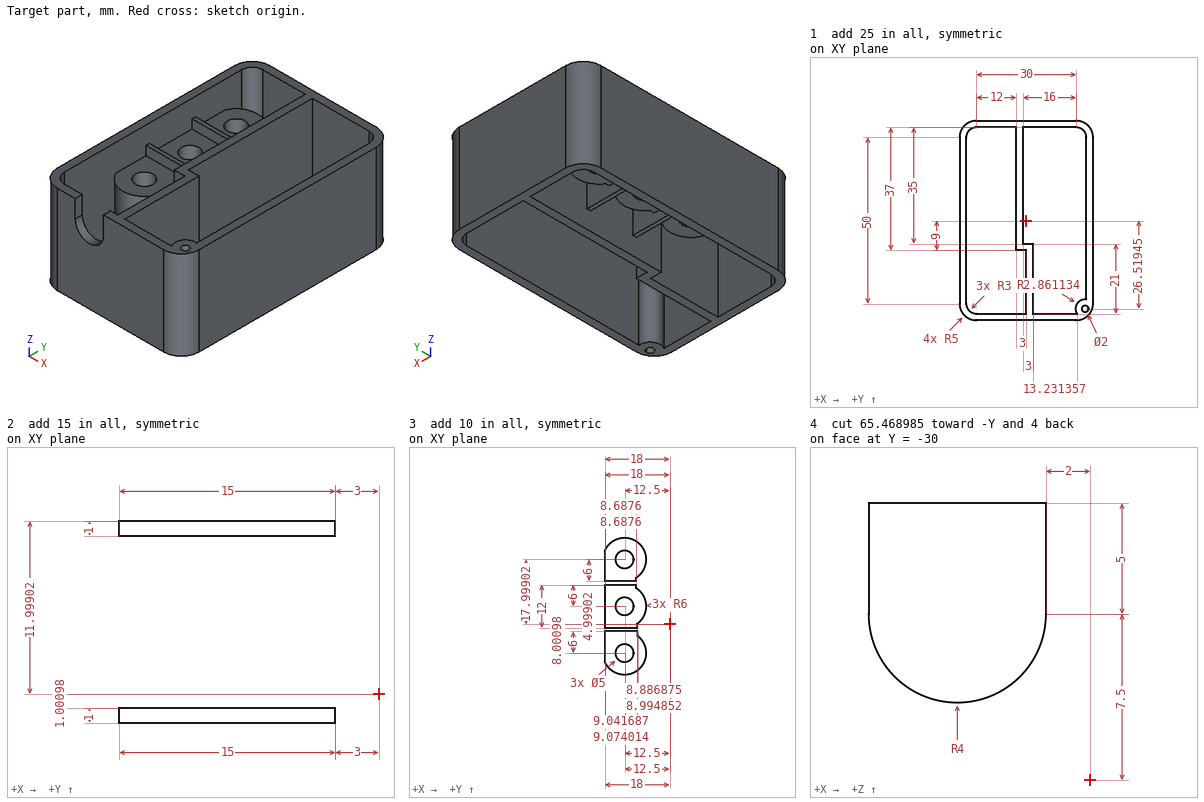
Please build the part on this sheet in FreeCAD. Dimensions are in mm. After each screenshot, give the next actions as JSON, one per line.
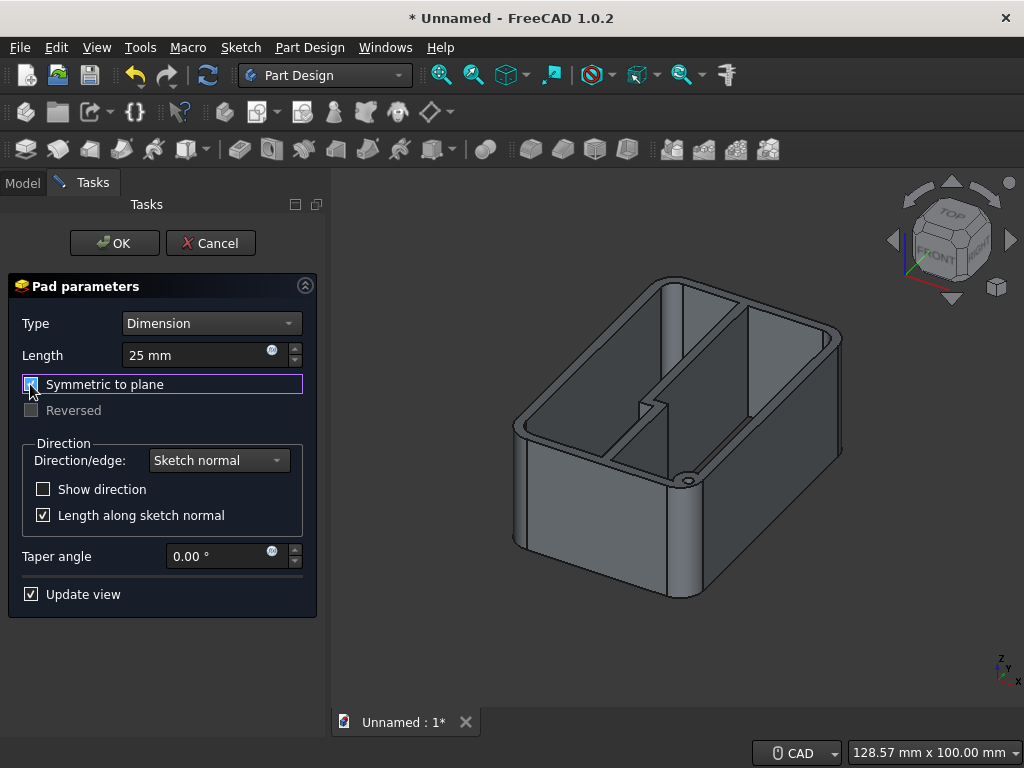
{"action": "left_click", "coordinate": [115, 243]}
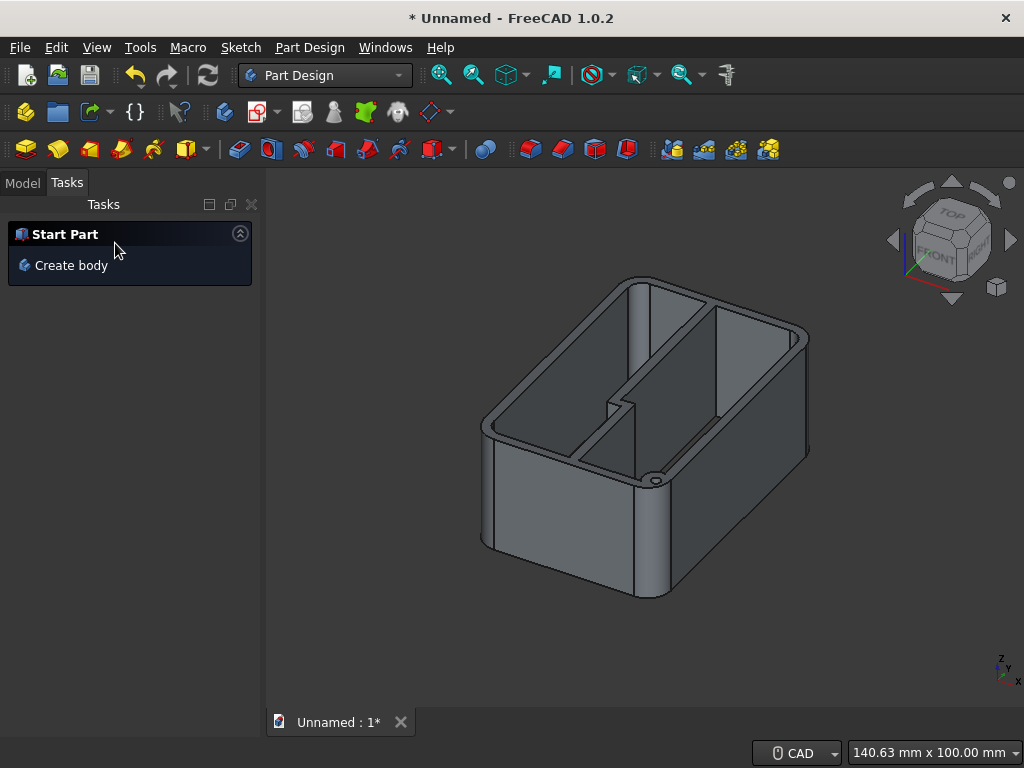
{"action": "left_click", "coordinate": [258, 112]}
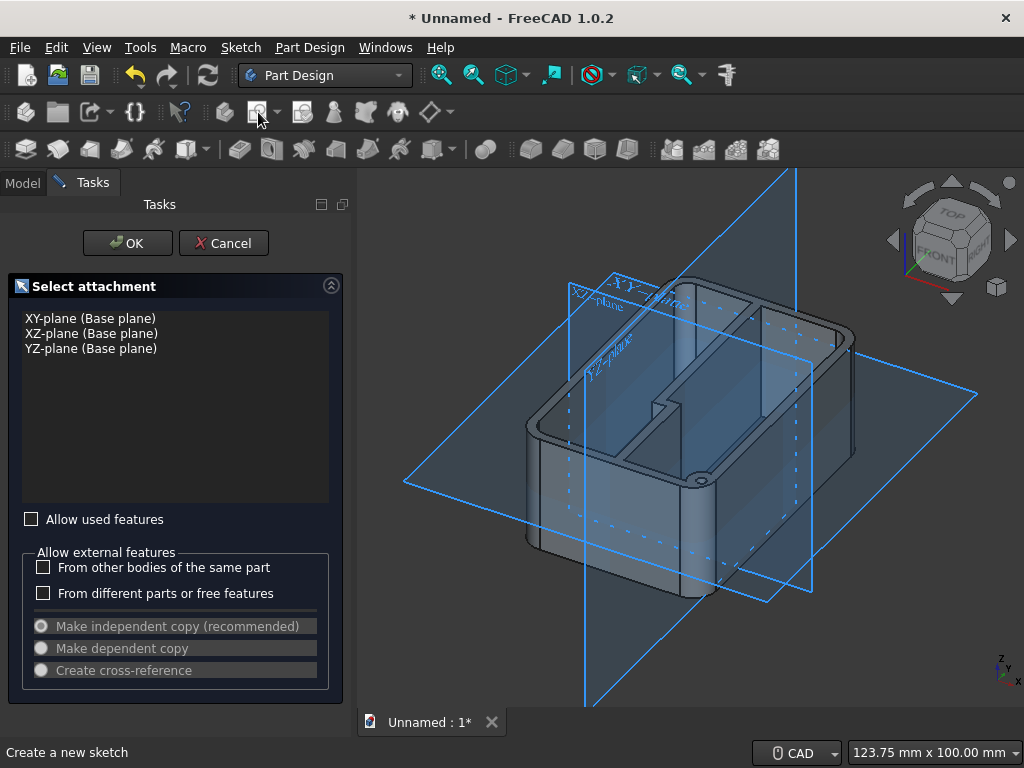
{"action": "left_click", "coordinate": [82, 318]}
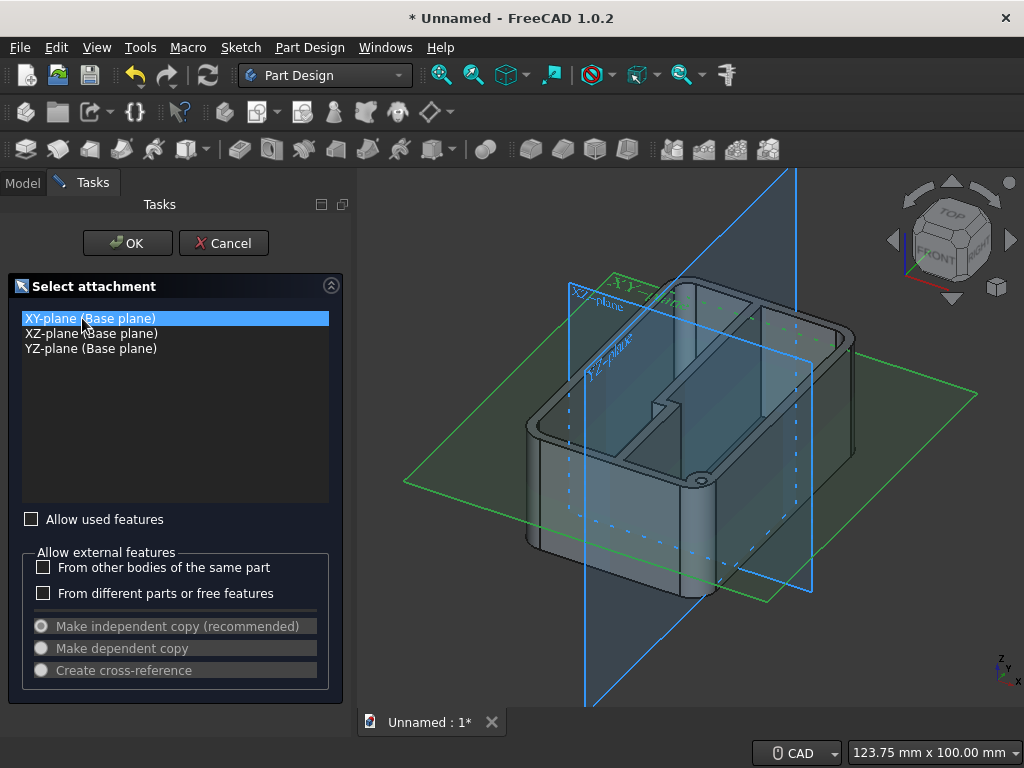
{"action": "left_click", "coordinate": [128, 243]}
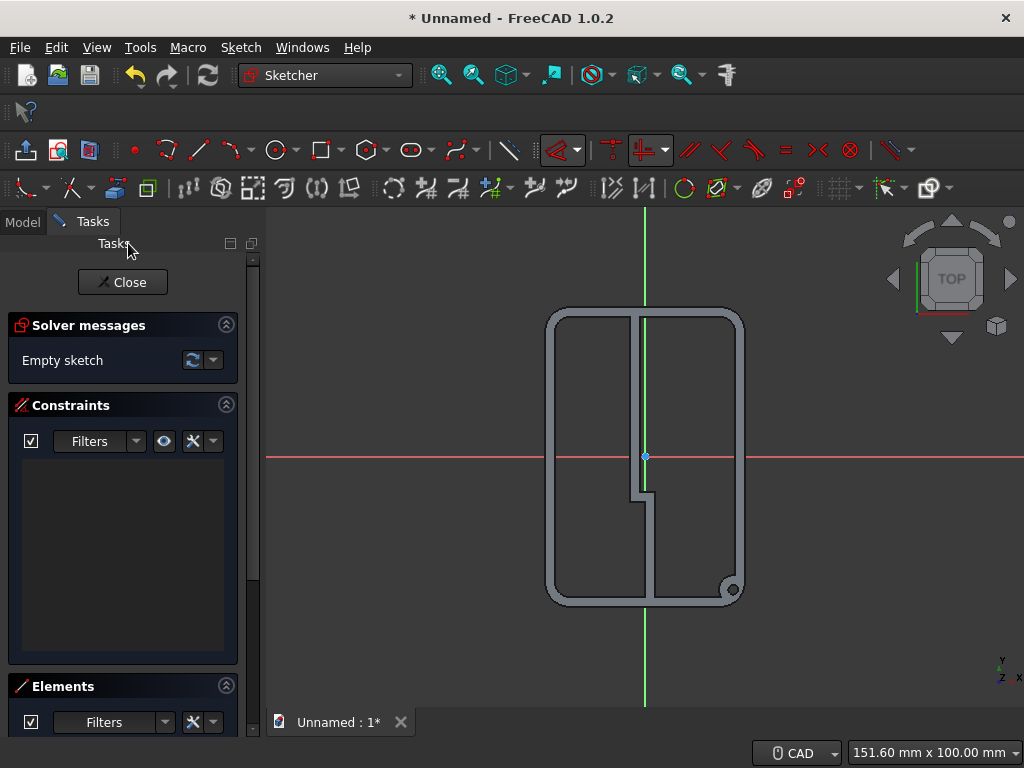
{"action": "left_click", "coordinate": [90, 150]}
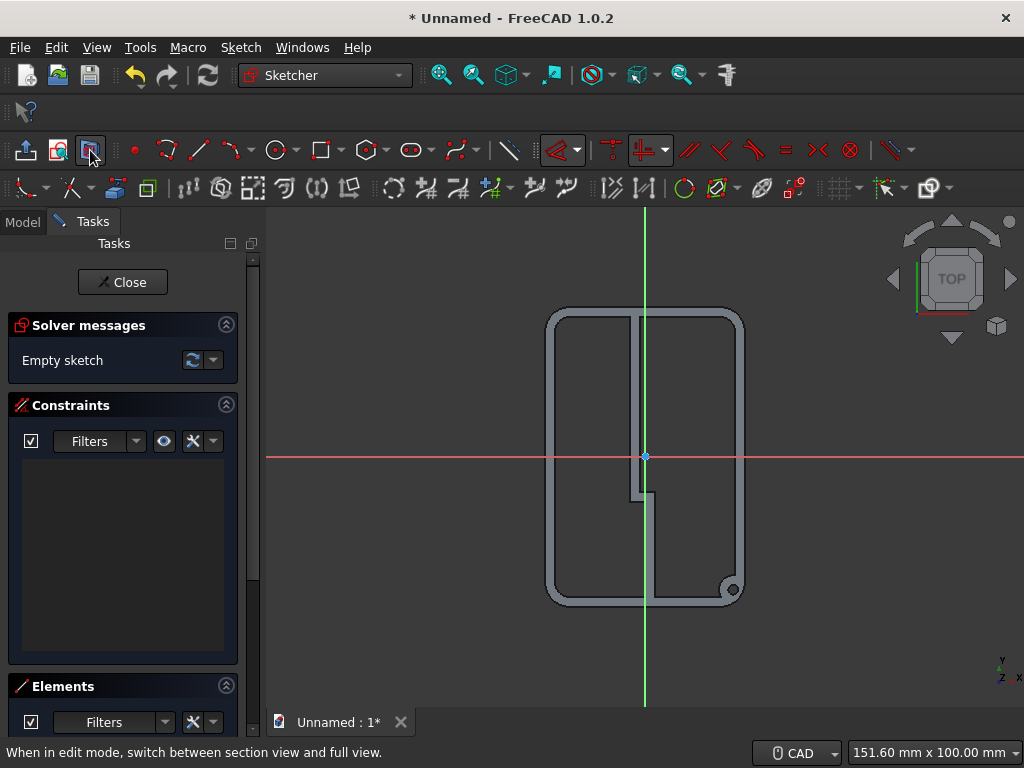
{"action": "scroll", "coordinate": [608, 424], "scroll_direction": "up", "scroll_amount": 7}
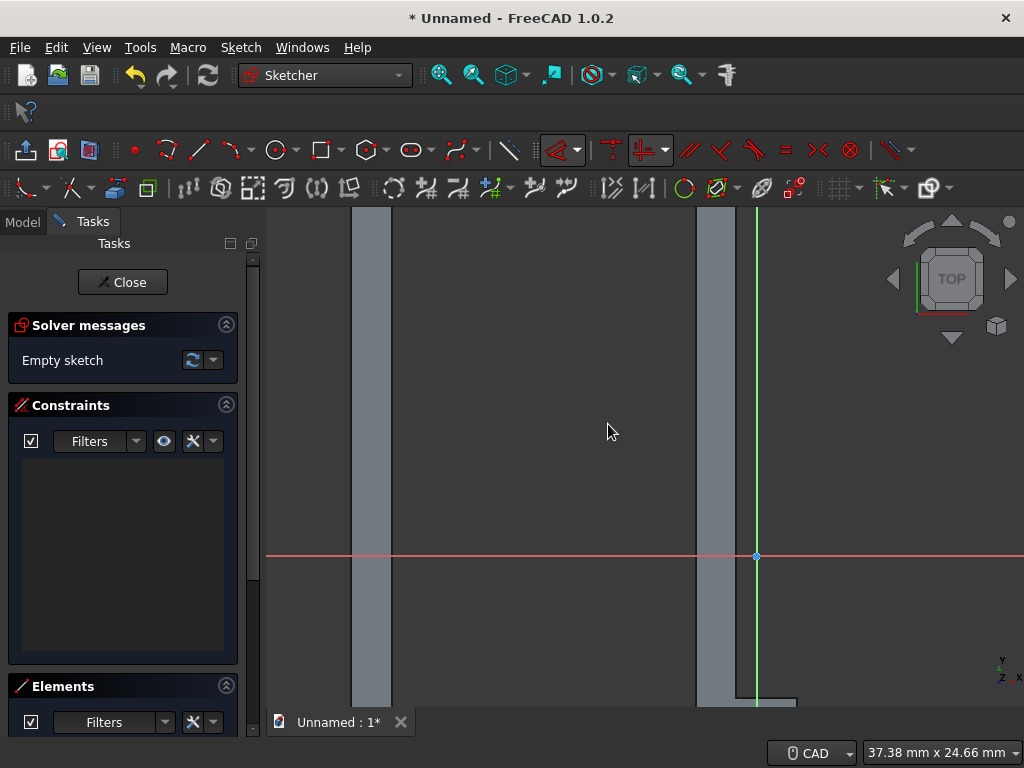
{"action": "left_click", "coordinate": [322, 150]}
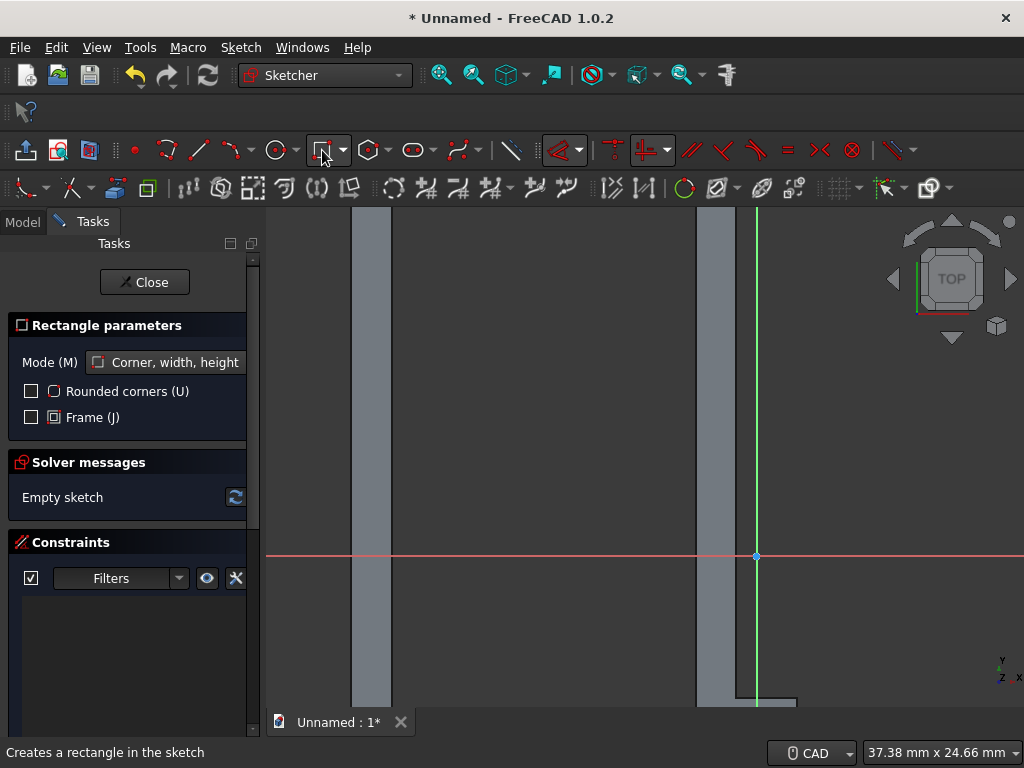
{"action": "left_click", "coordinate": [392, 577]}
{"action": "left_click", "coordinate": [696, 597]}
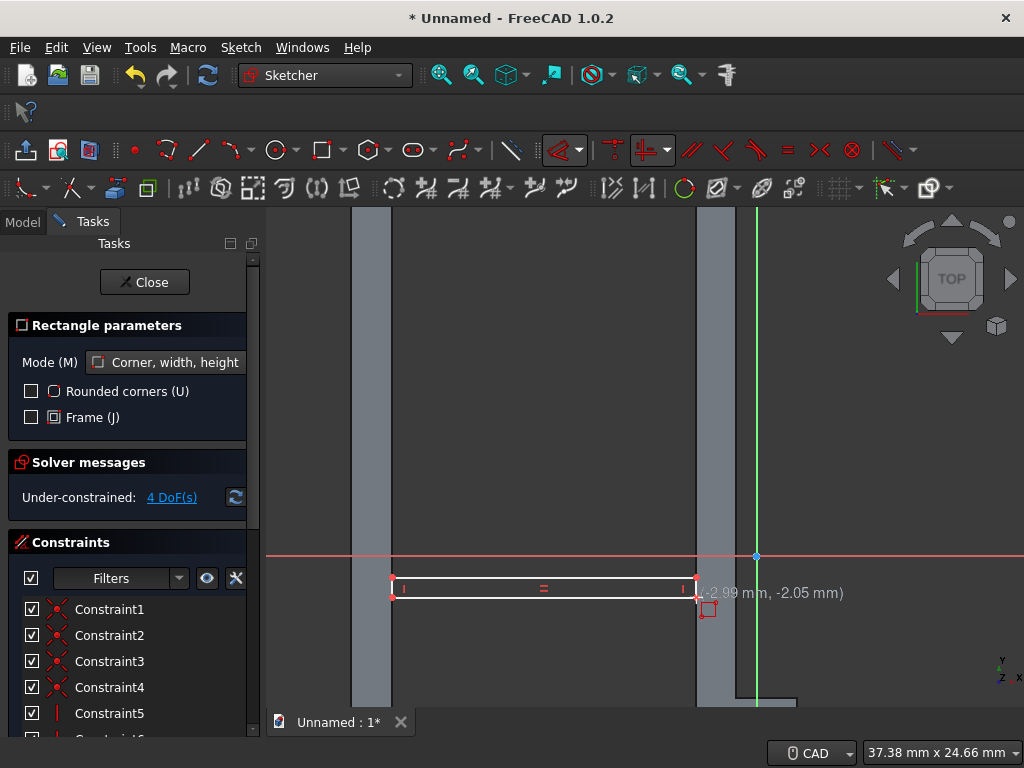
{"action": "left_click", "coordinate": [392, 313]}
{"action": "left_click", "coordinate": [696, 333]}
{"action": "key", "text": "Escape"}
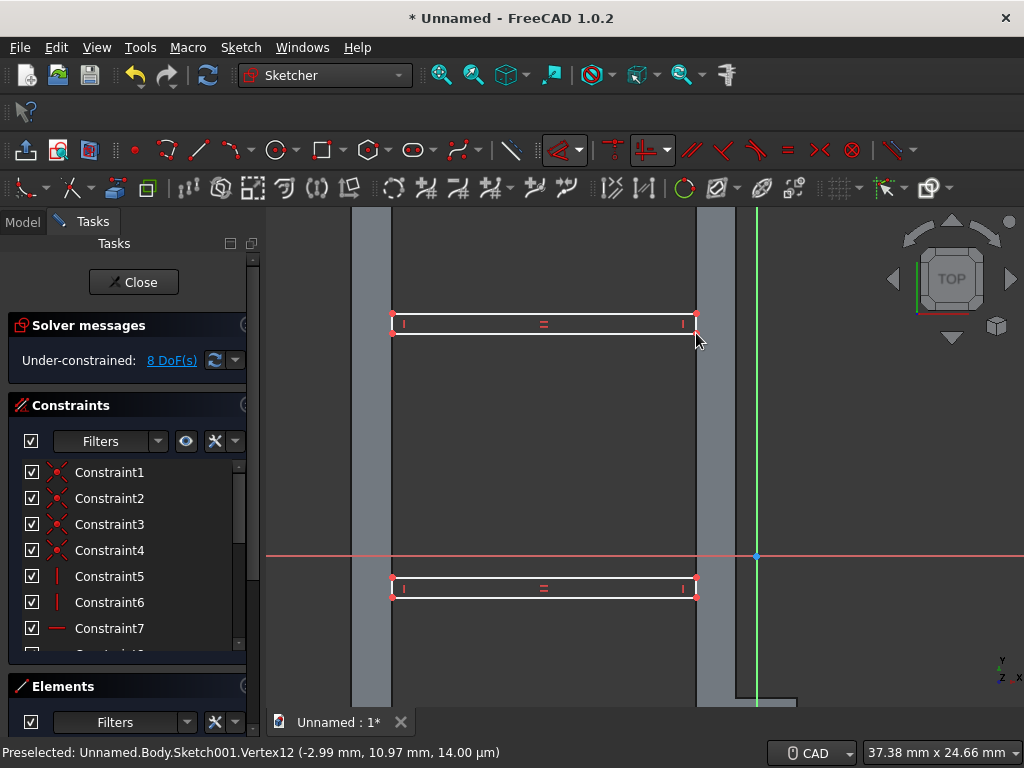
{"action": "scroll", "coordinate": [392, 588], "scroll_direction": "up", "scroll_amount": 4}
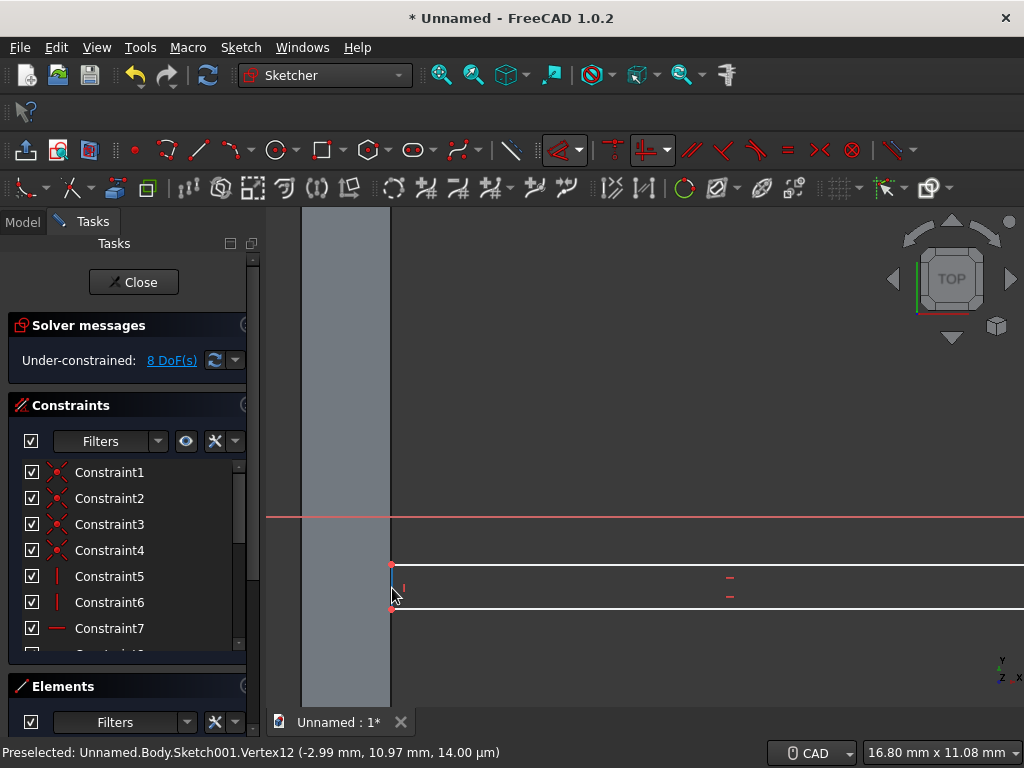
{"action": "left_click", "coordinate": [392, 587]}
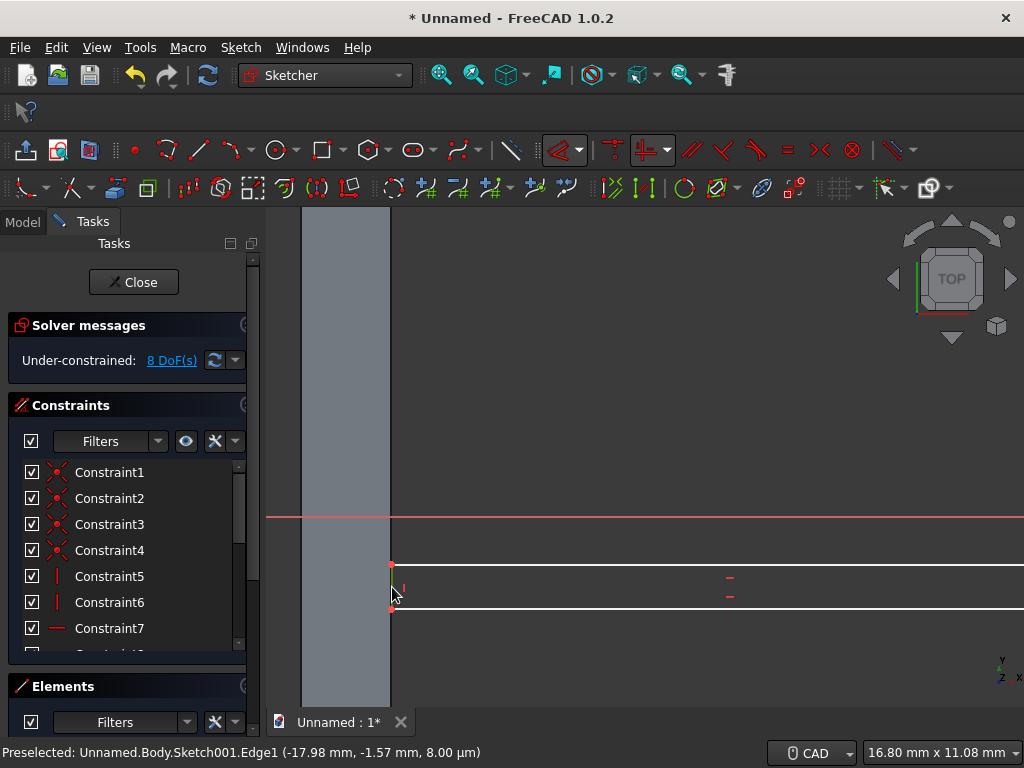
{"action": "left_click", "coordinate": [582, 150]}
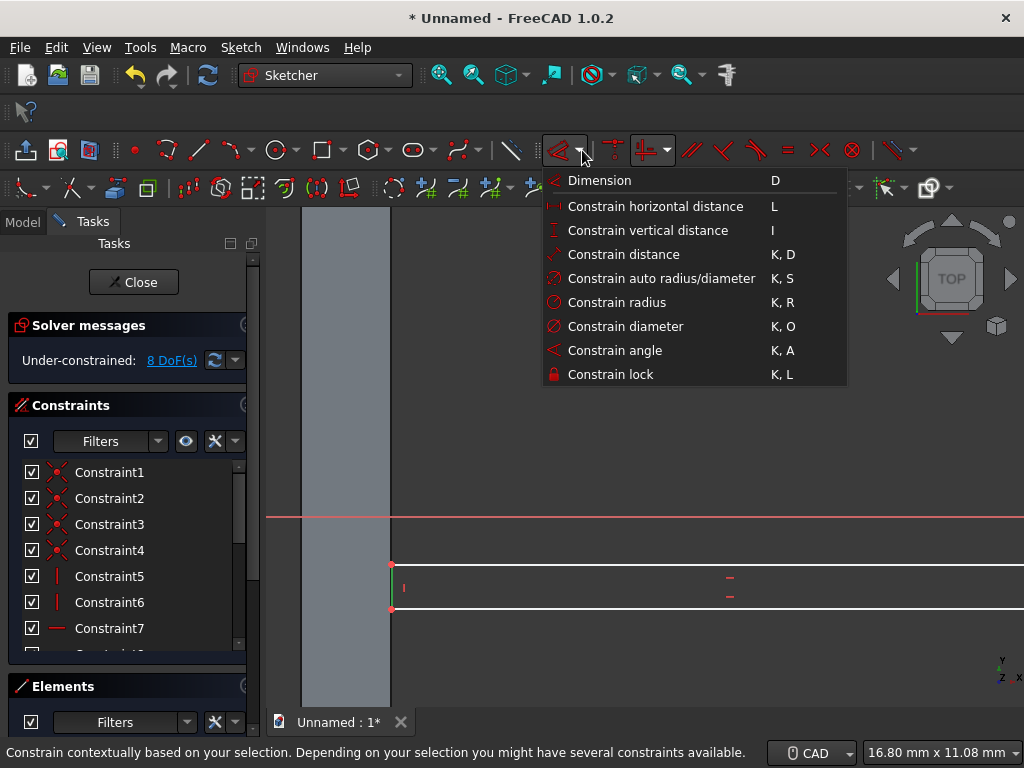
{"action": "left_click", "coordinate": [695, 230]}